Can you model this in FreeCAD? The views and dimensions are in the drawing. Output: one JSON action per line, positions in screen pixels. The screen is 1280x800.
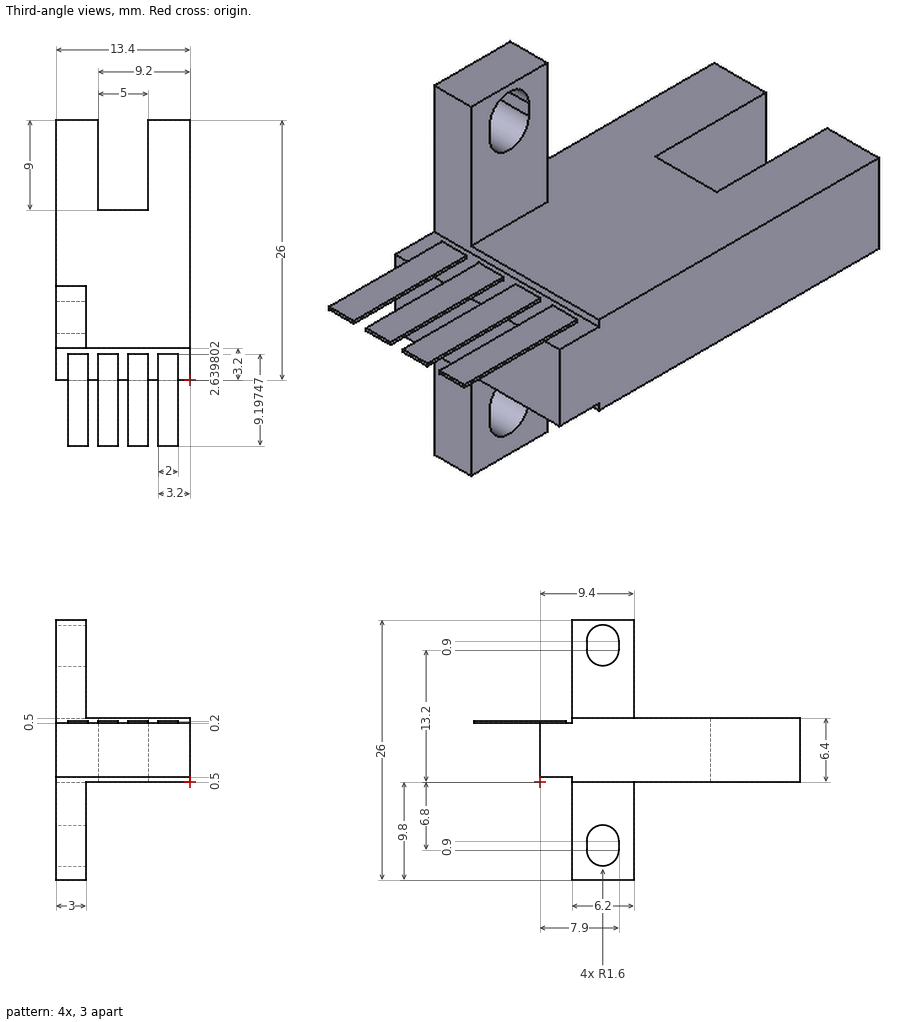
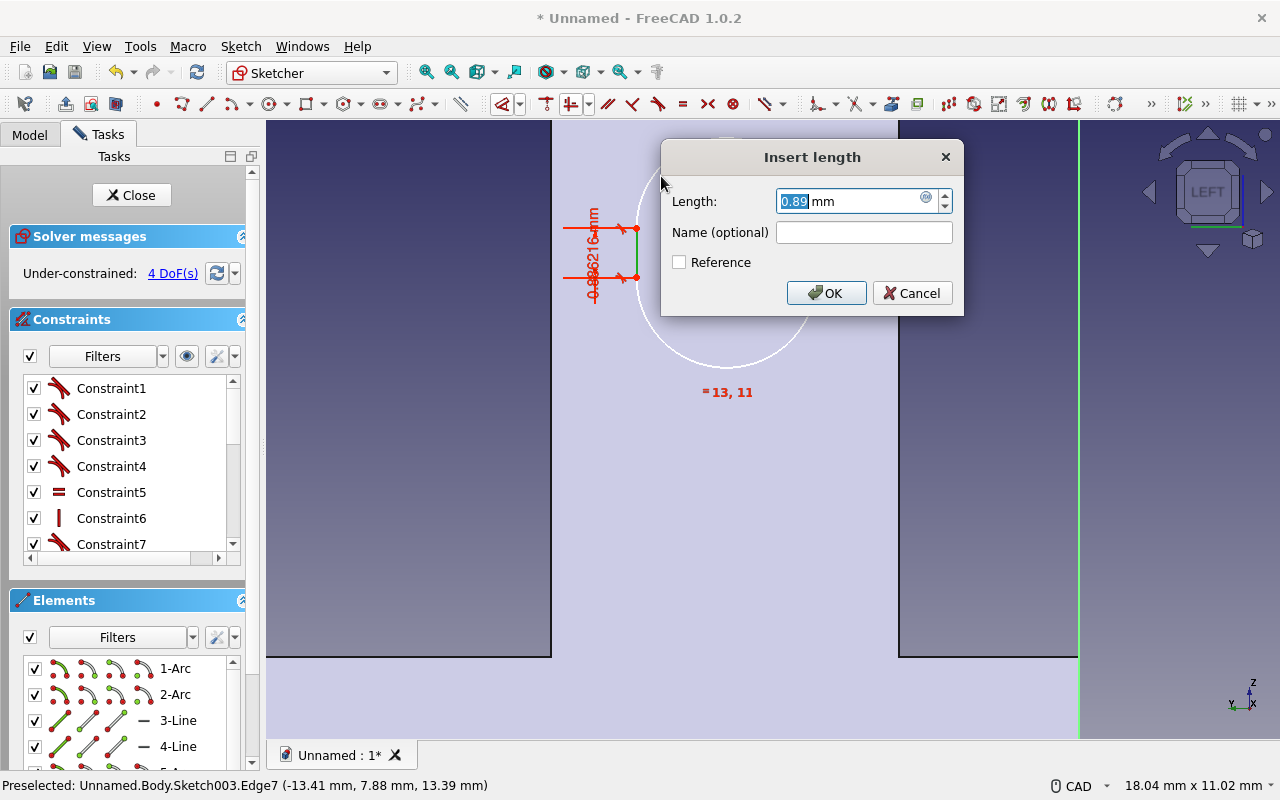
{"action": "type", "text": "0.9"}
{"action": "key", "text": "Return"}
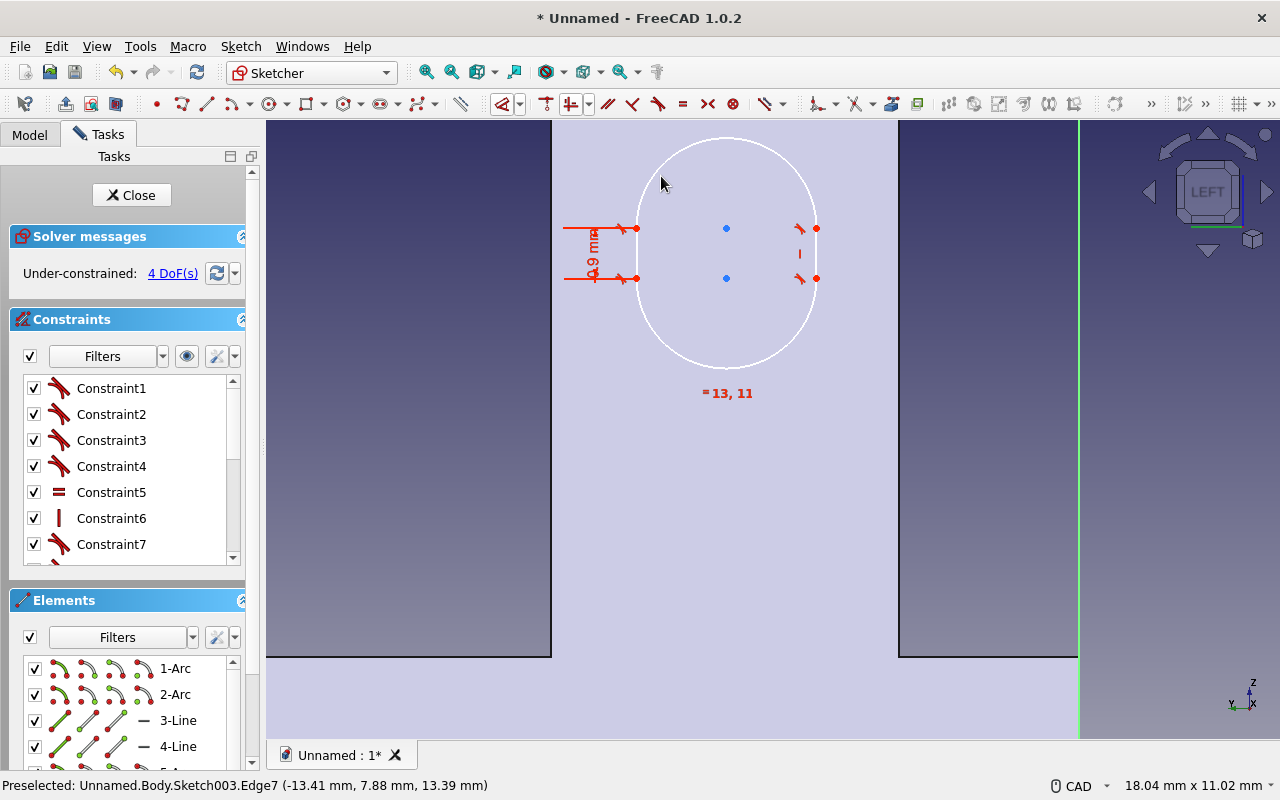
{"action": "scroll", "coordinate": [639, 265], "scroll_direction": "down", "scroll_amount": 6}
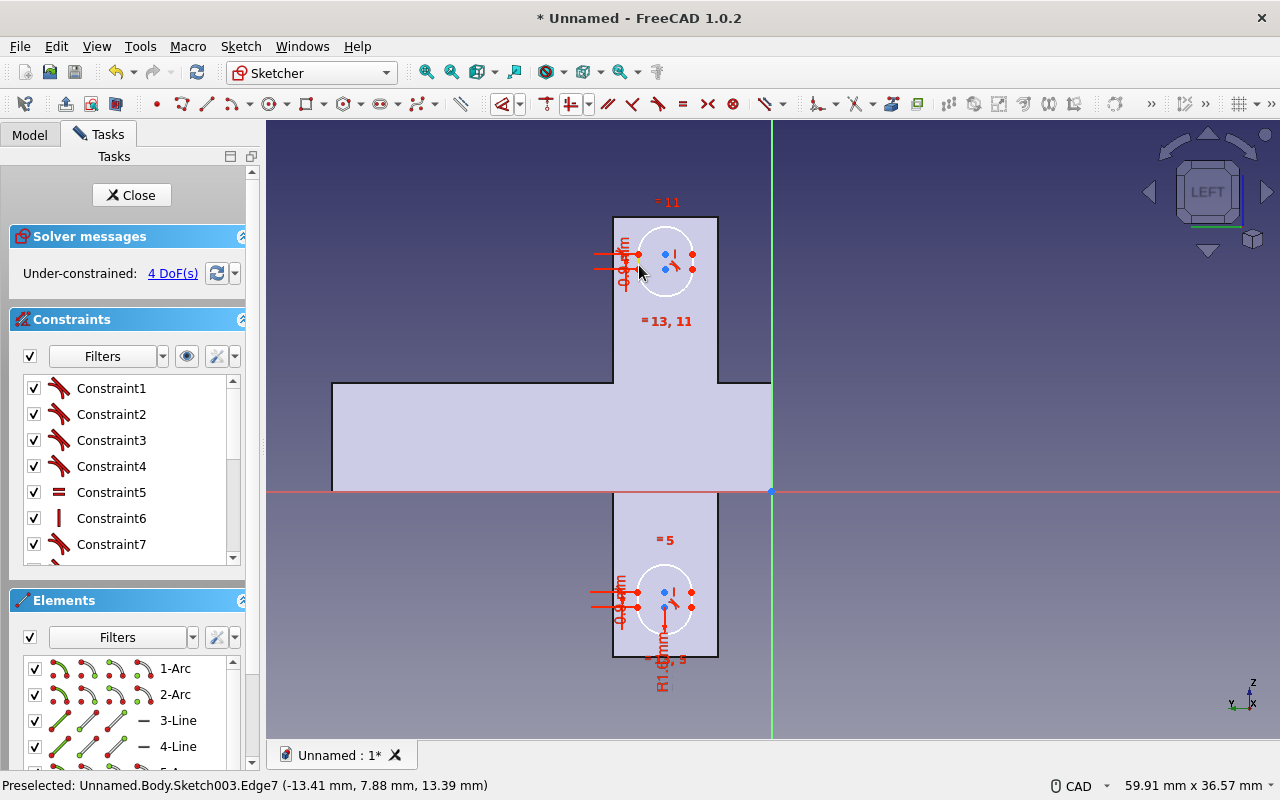
{"action": "left_click", "coordinate": [638, 607]}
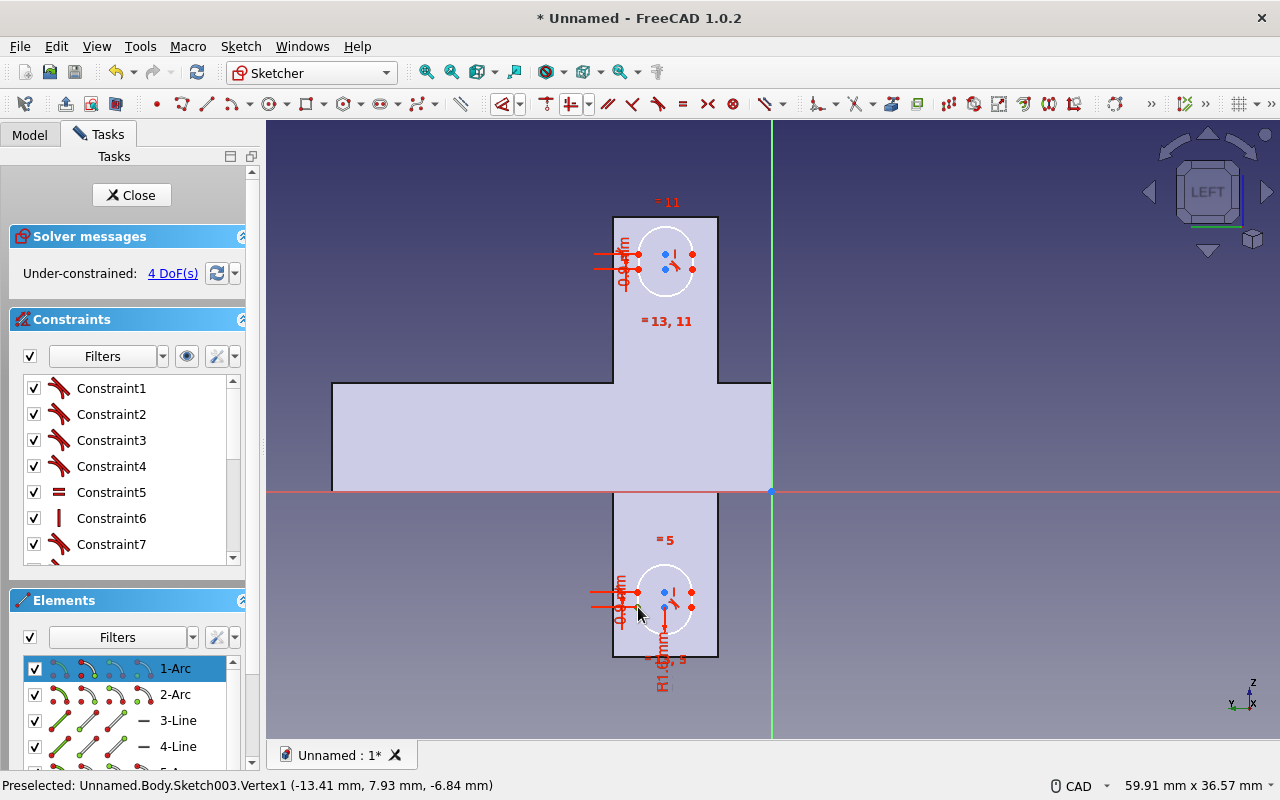
{"action": "left_click", "coordinate": [520, 104]}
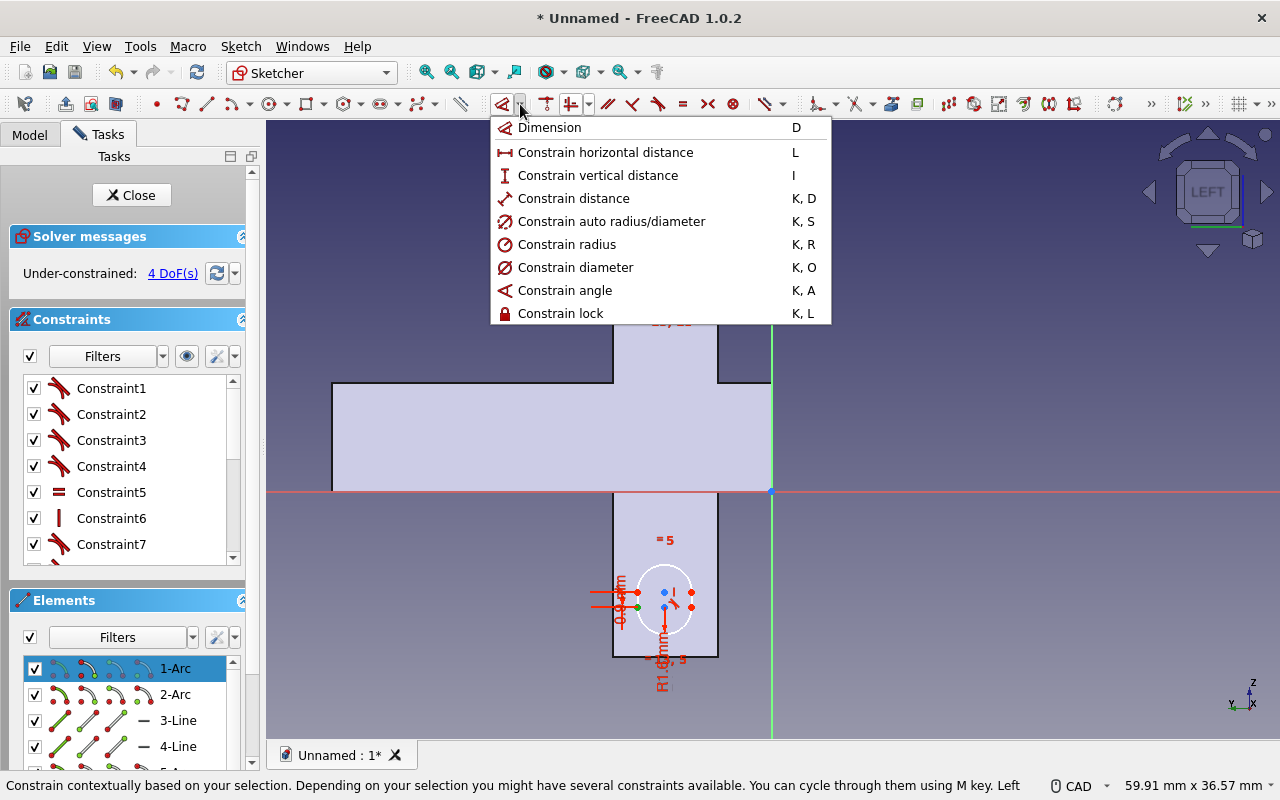
{"action": "left_click", "coordinate": [661, 152]}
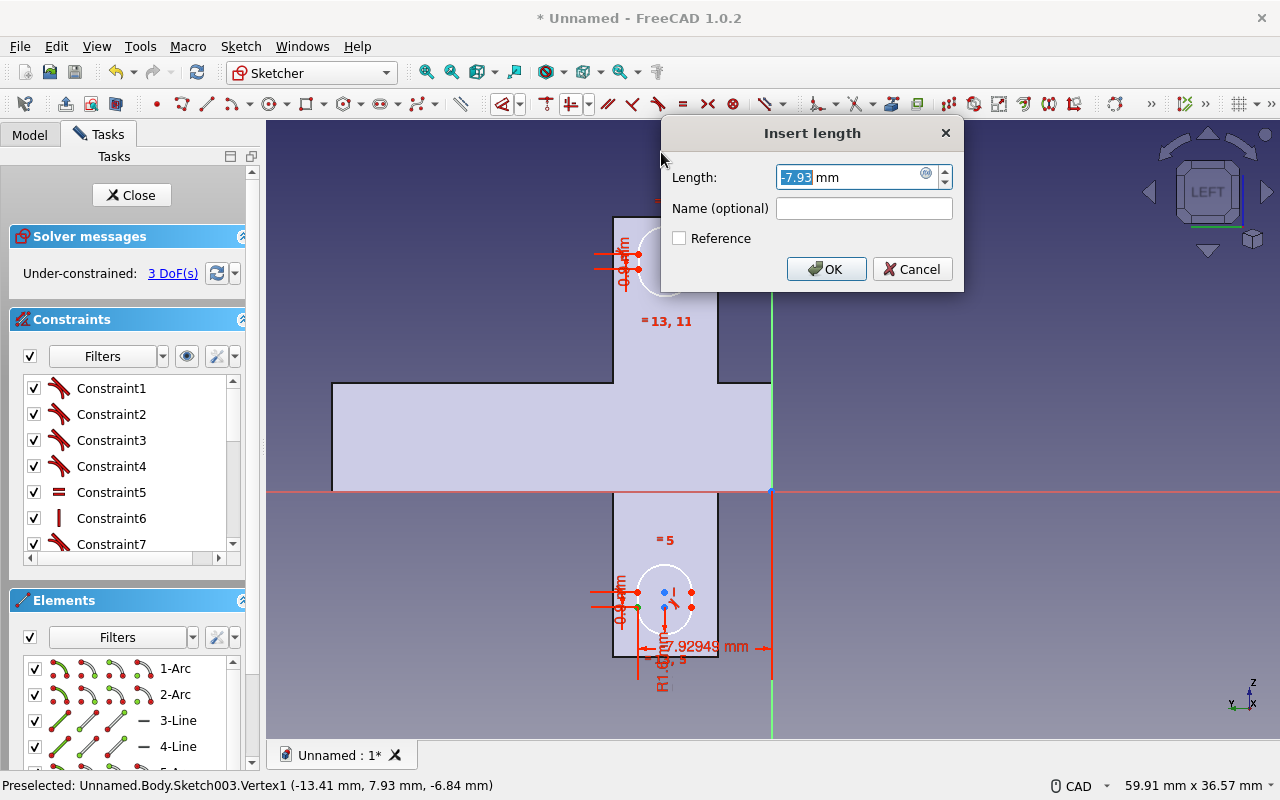
{"action": "type", "text": "-7.9"}
{"action": "key", "text": "Return"}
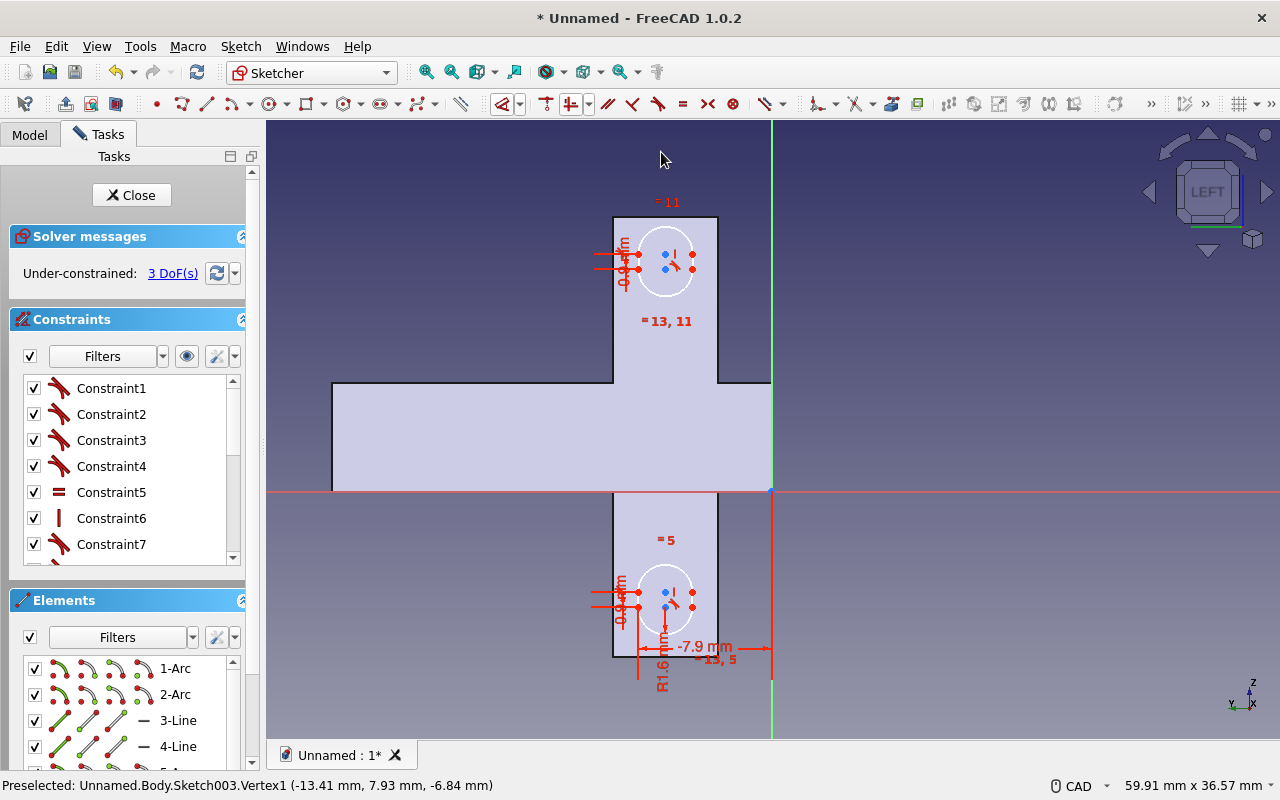
{"action": "left_click", "coordinate": [638, 607]}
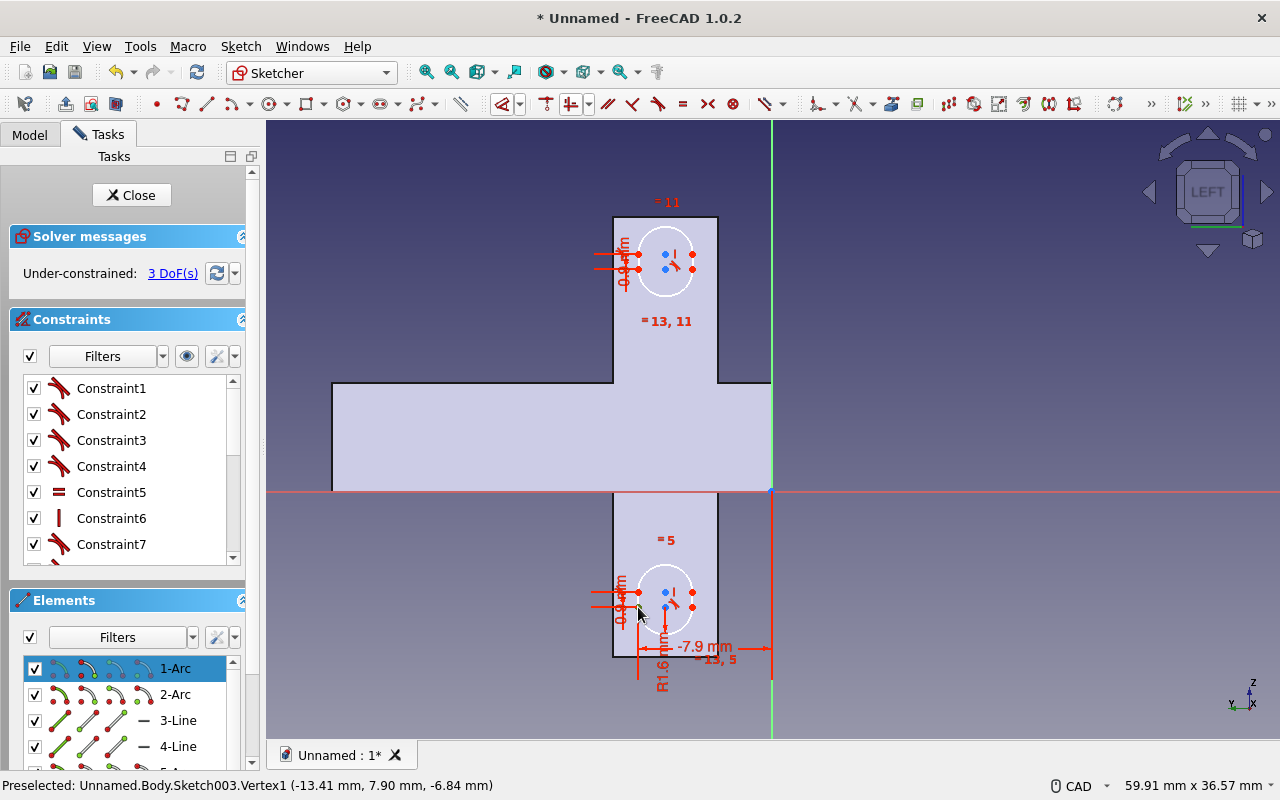
{"action": "key", "text": "i"}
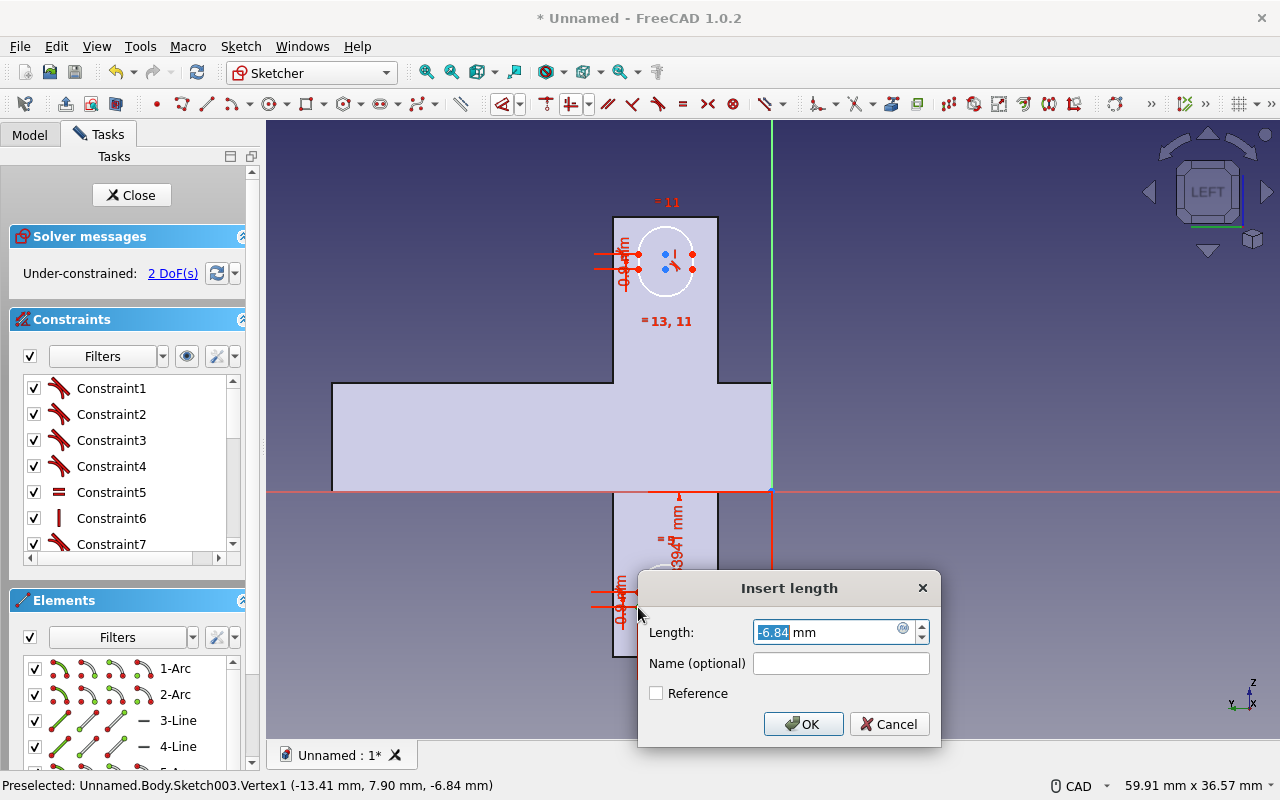
{"action": "type", "text": "-6.8"}
{"action": "key", "text": "Return"}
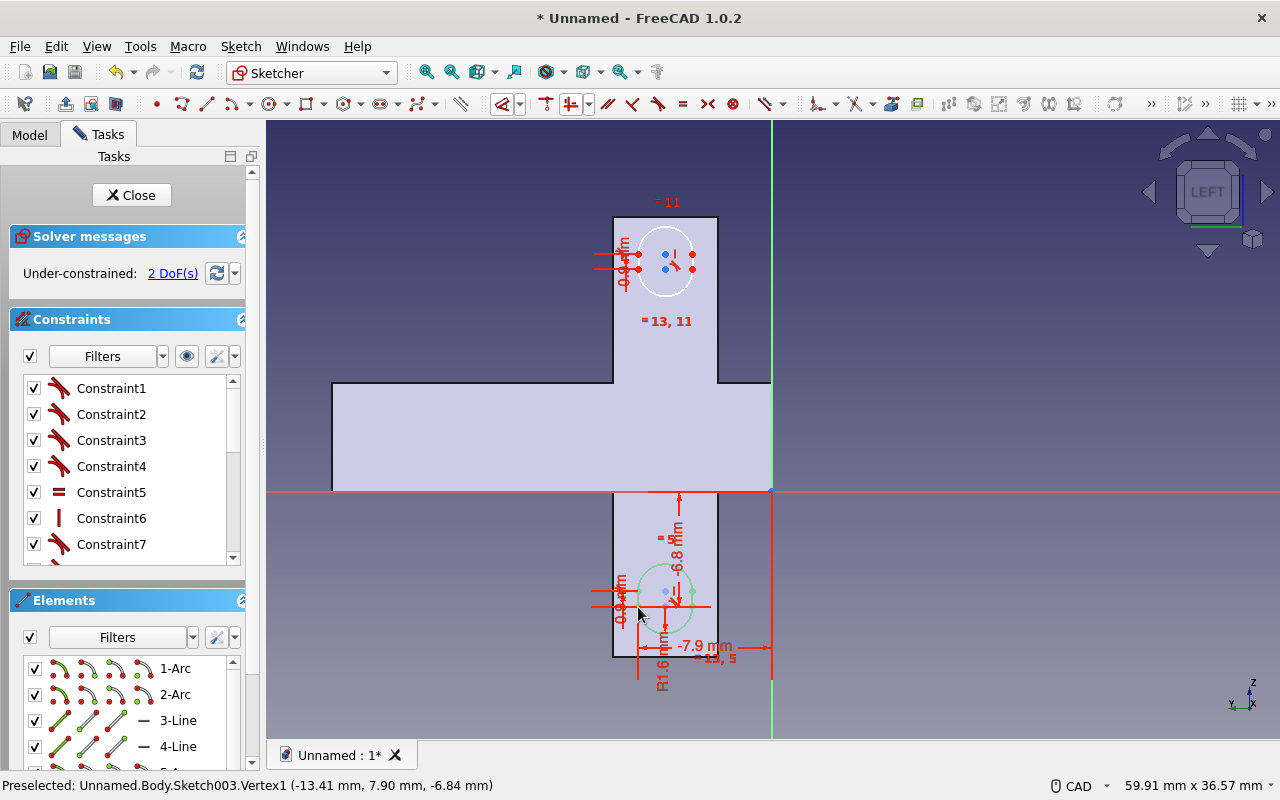
{"action": "left_click", "coordinate": [639, 269]}